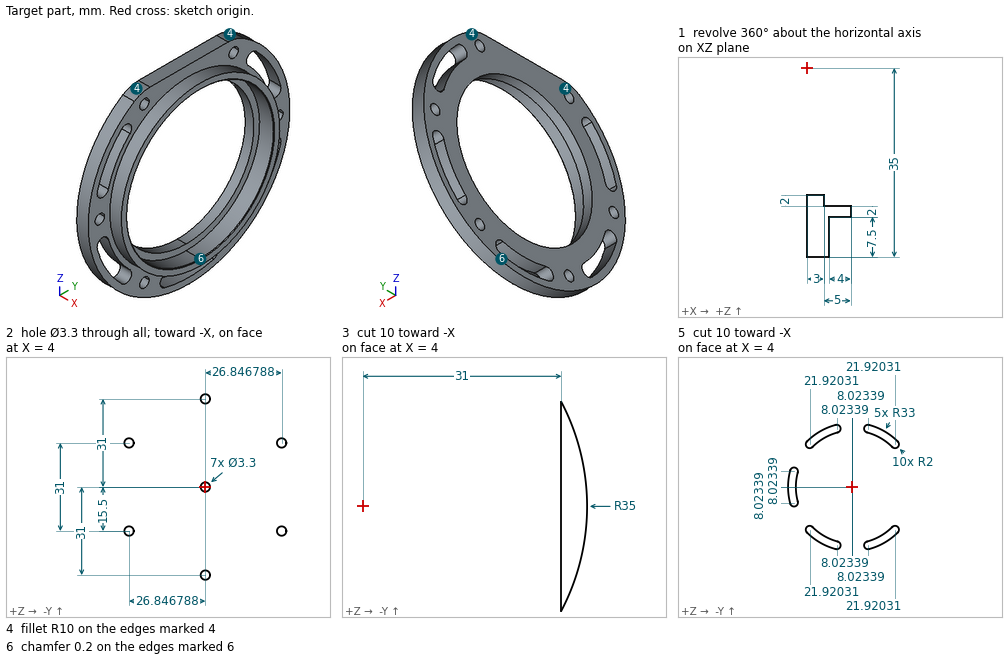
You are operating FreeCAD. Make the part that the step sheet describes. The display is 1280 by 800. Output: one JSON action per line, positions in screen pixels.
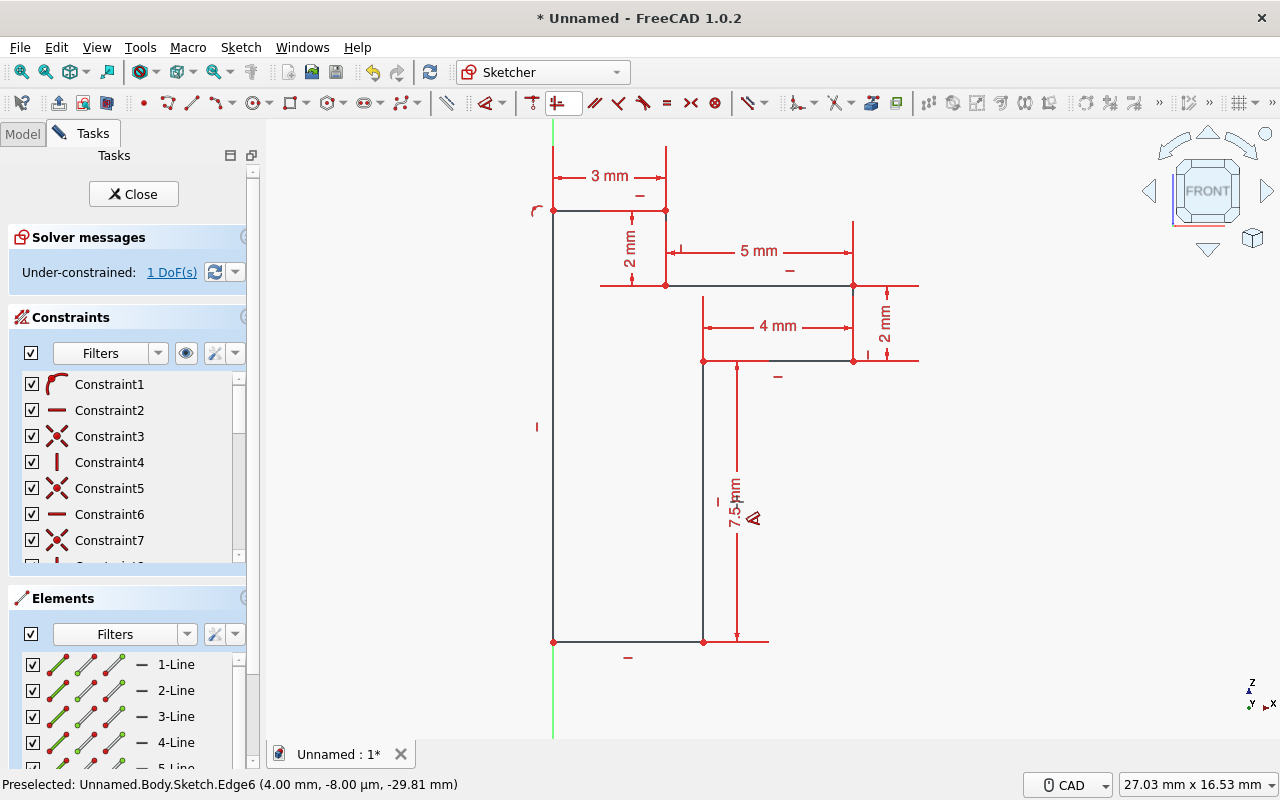
{"action": "left_click", "coordinate": [703, 642]}
{"action": "left_click", "coordinate": [519, 395]}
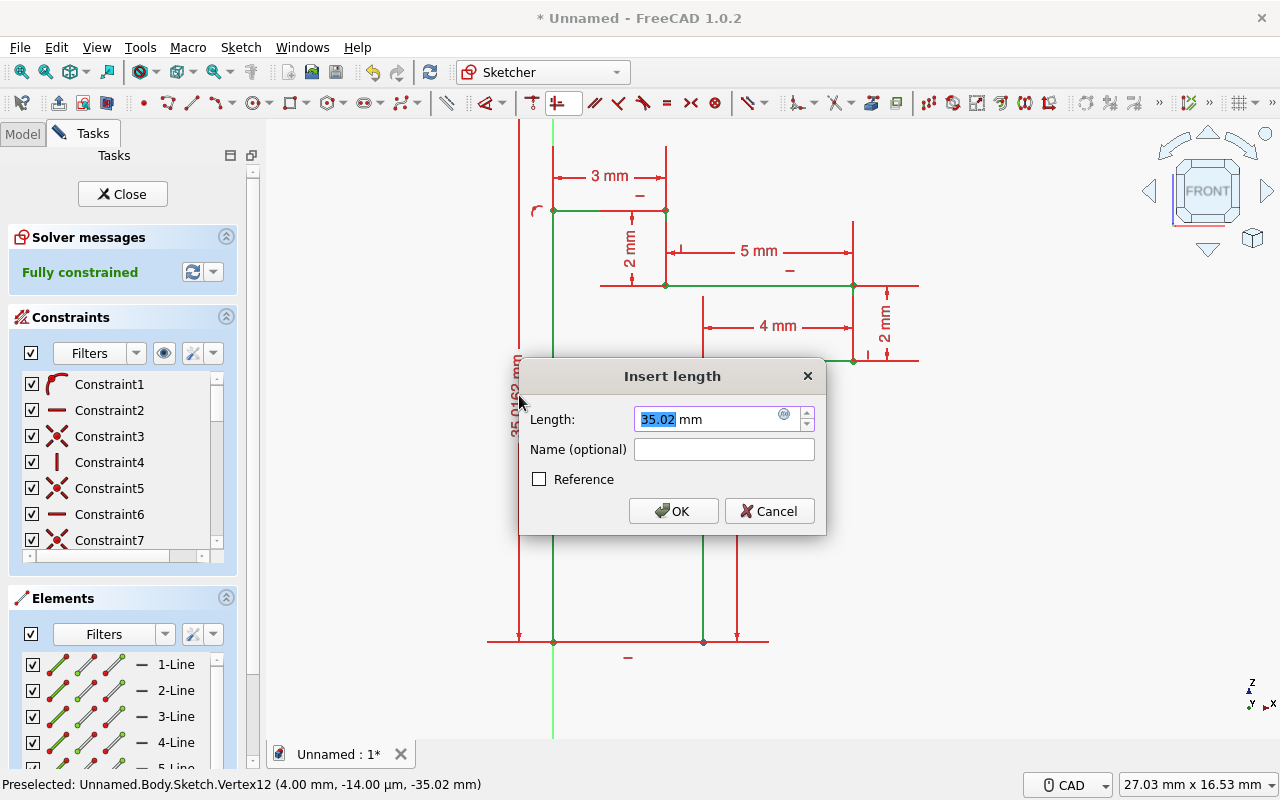
{"action": "type", "text": "35"}
{"action": "key", "text": "Return"}
{"action": "key", "text": "Escape"}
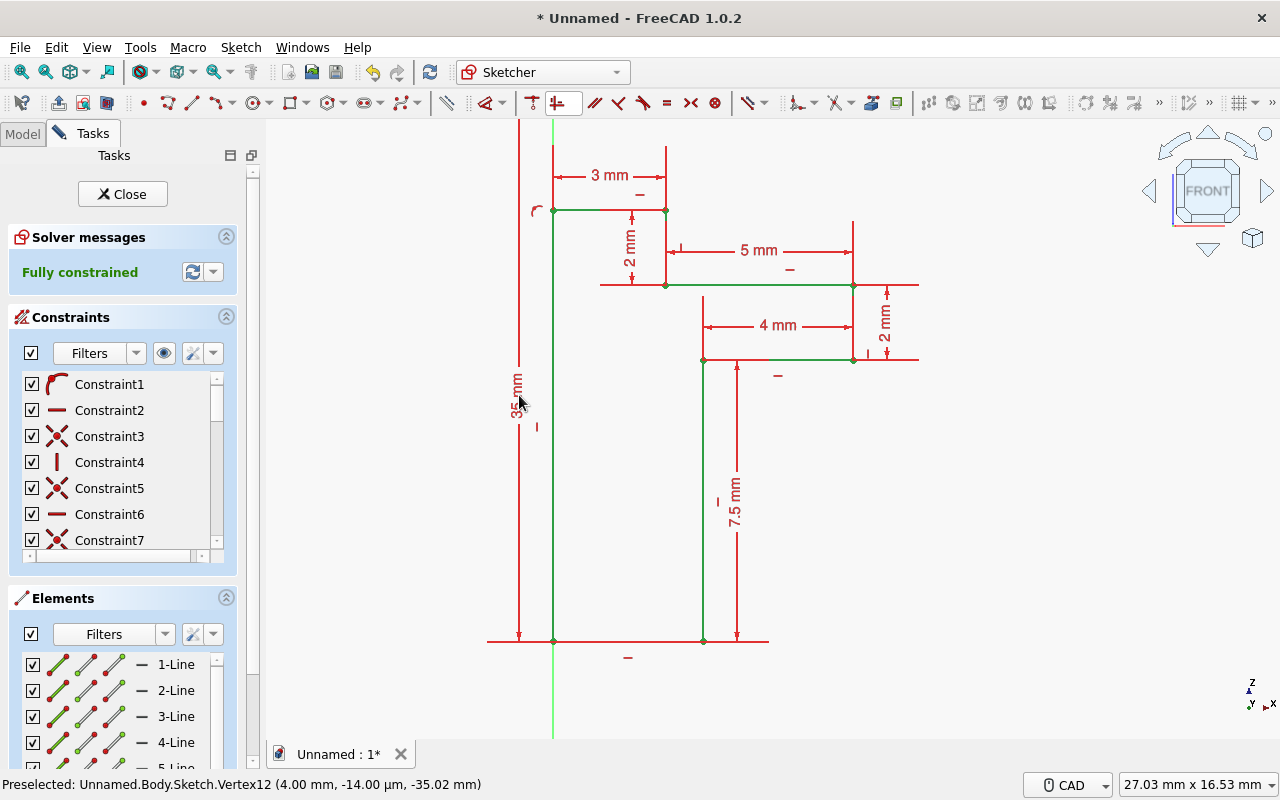
{"action": "left_click", "coordinate": [123, 194]}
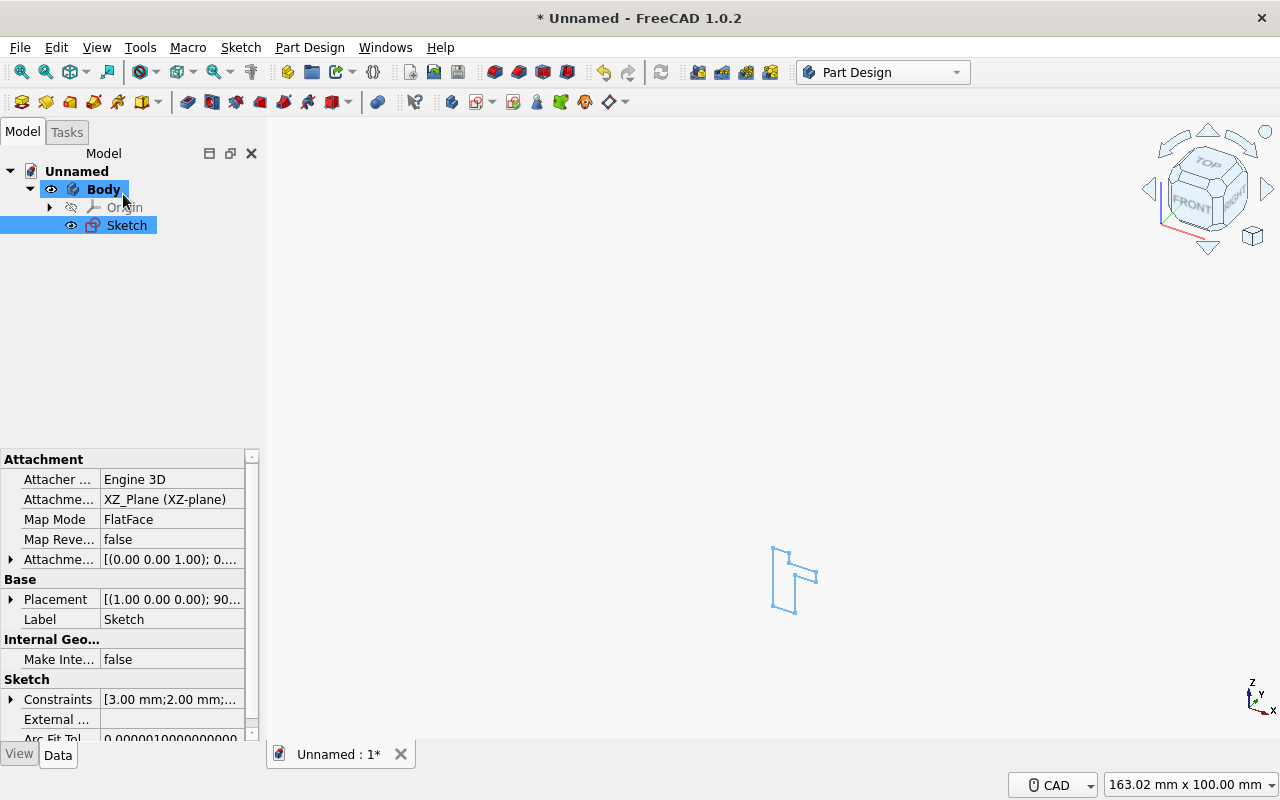
{"action": "left_click", "coordinate": [46, 102]}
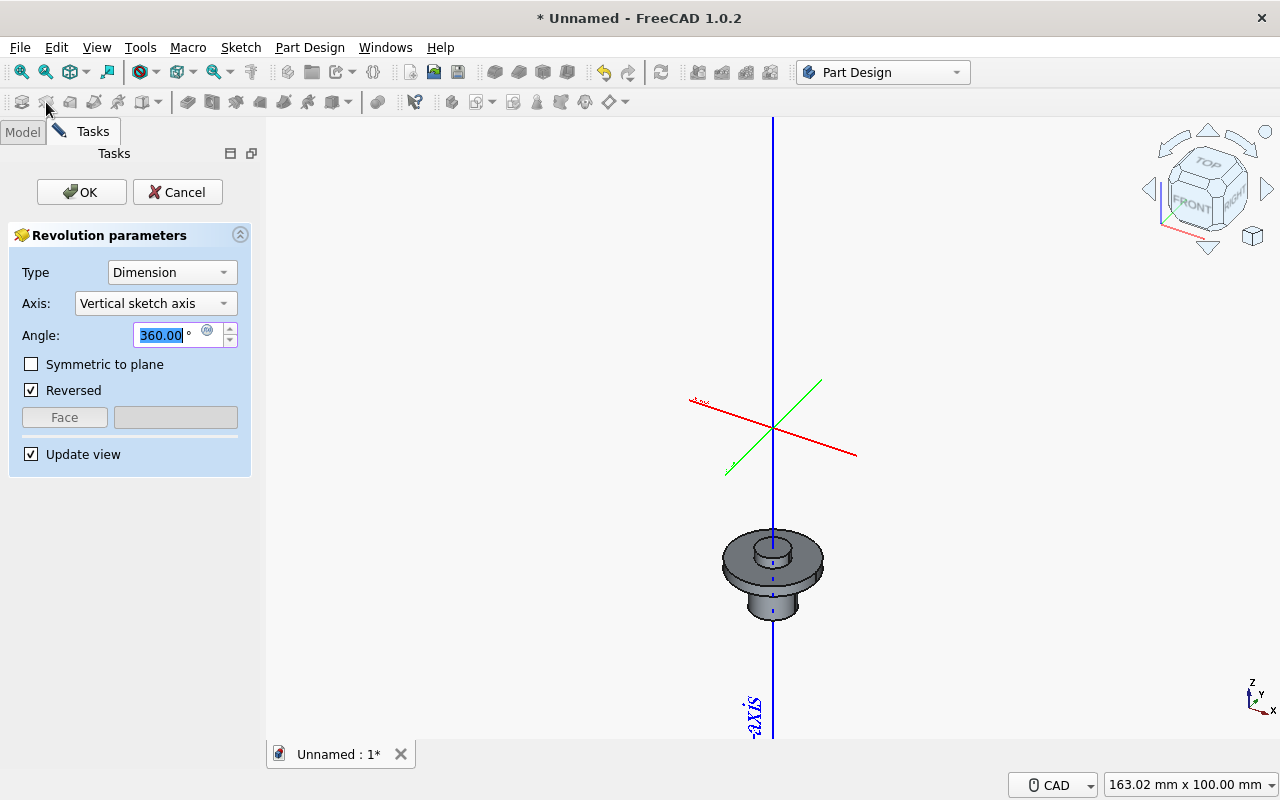
{"action": "left_click", "coordinate": [156, 304]}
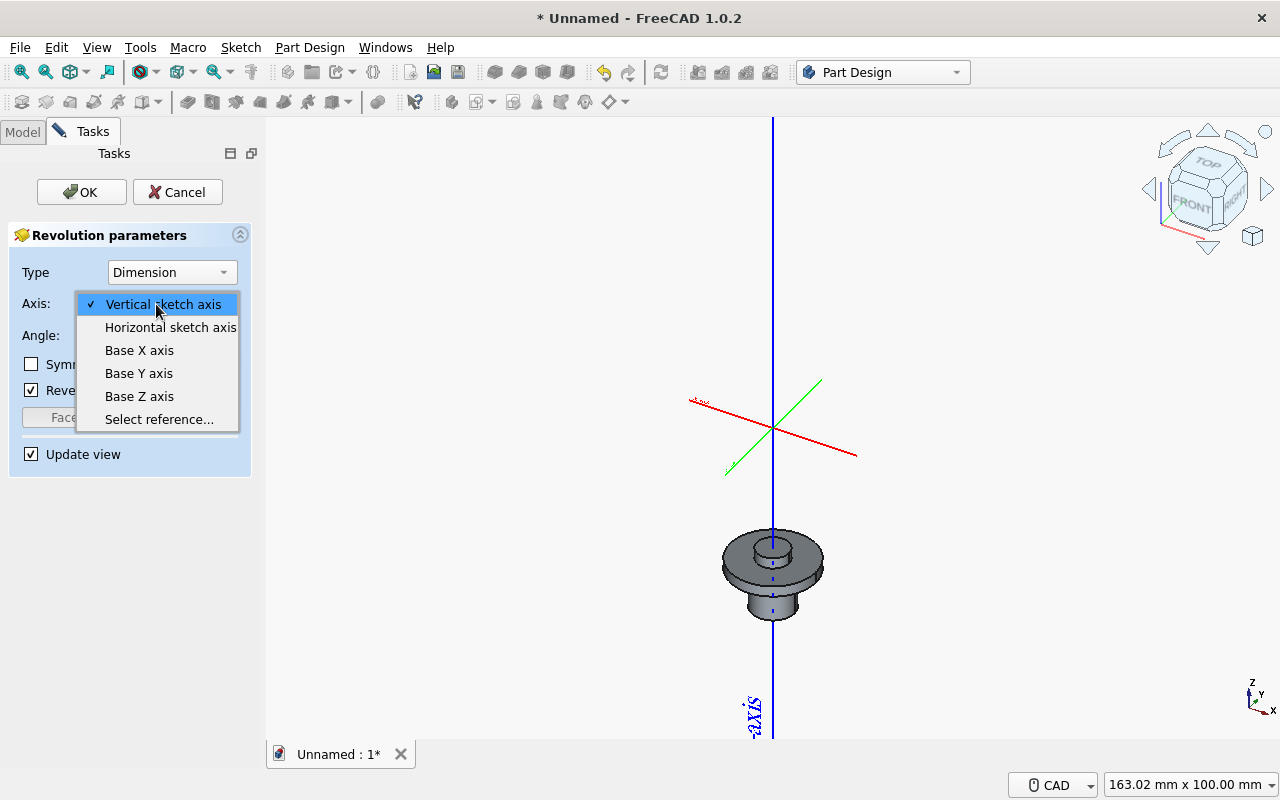
{"action": "left_click", "coordinate": [156, 328]}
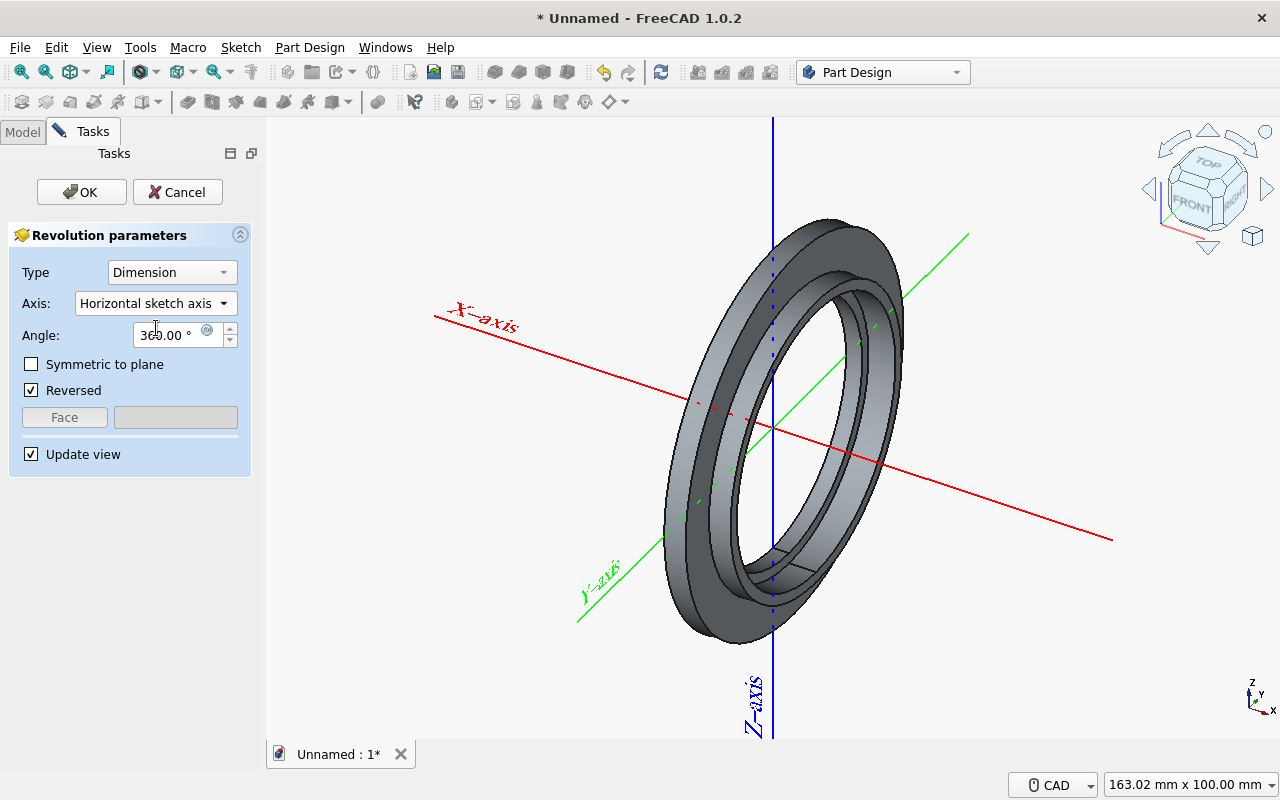
{"action": "left_click", "coordinate": [82, 192]}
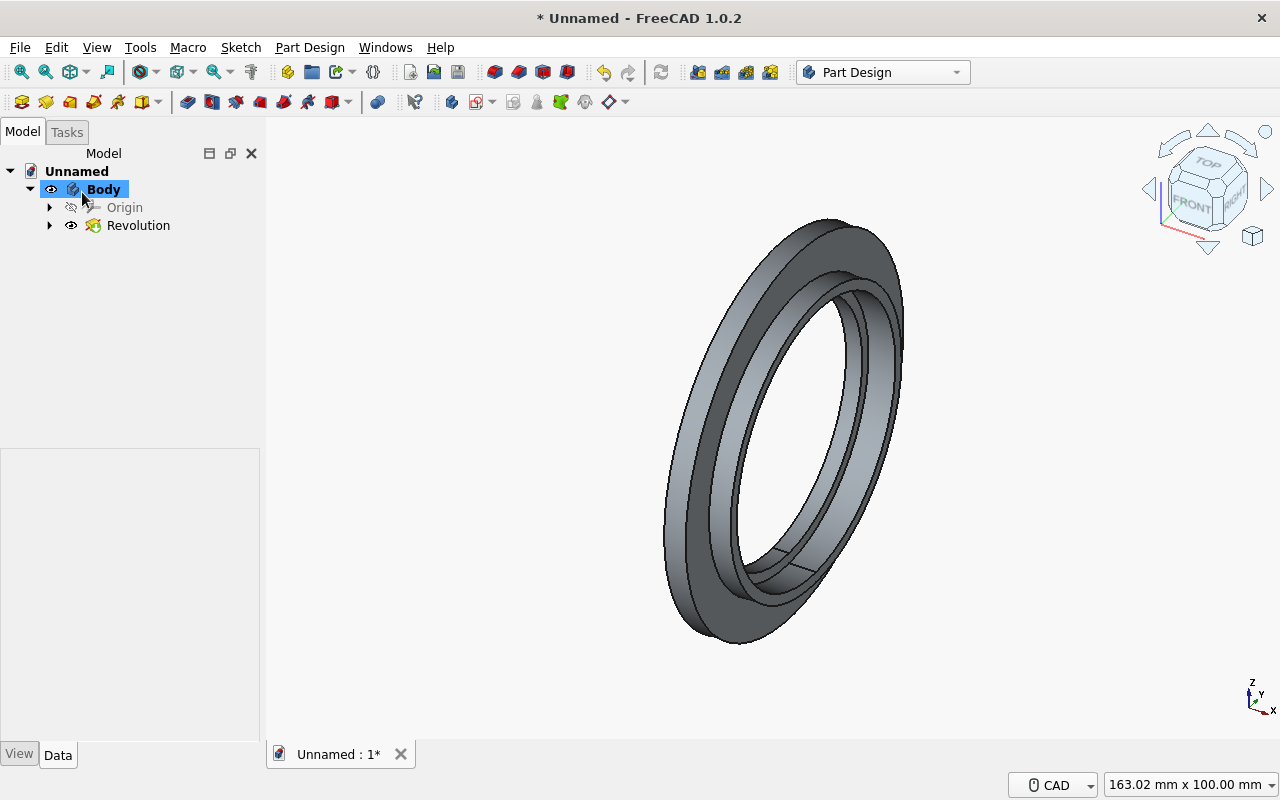
{"action": "left_click", "coordinate": [701, 476]}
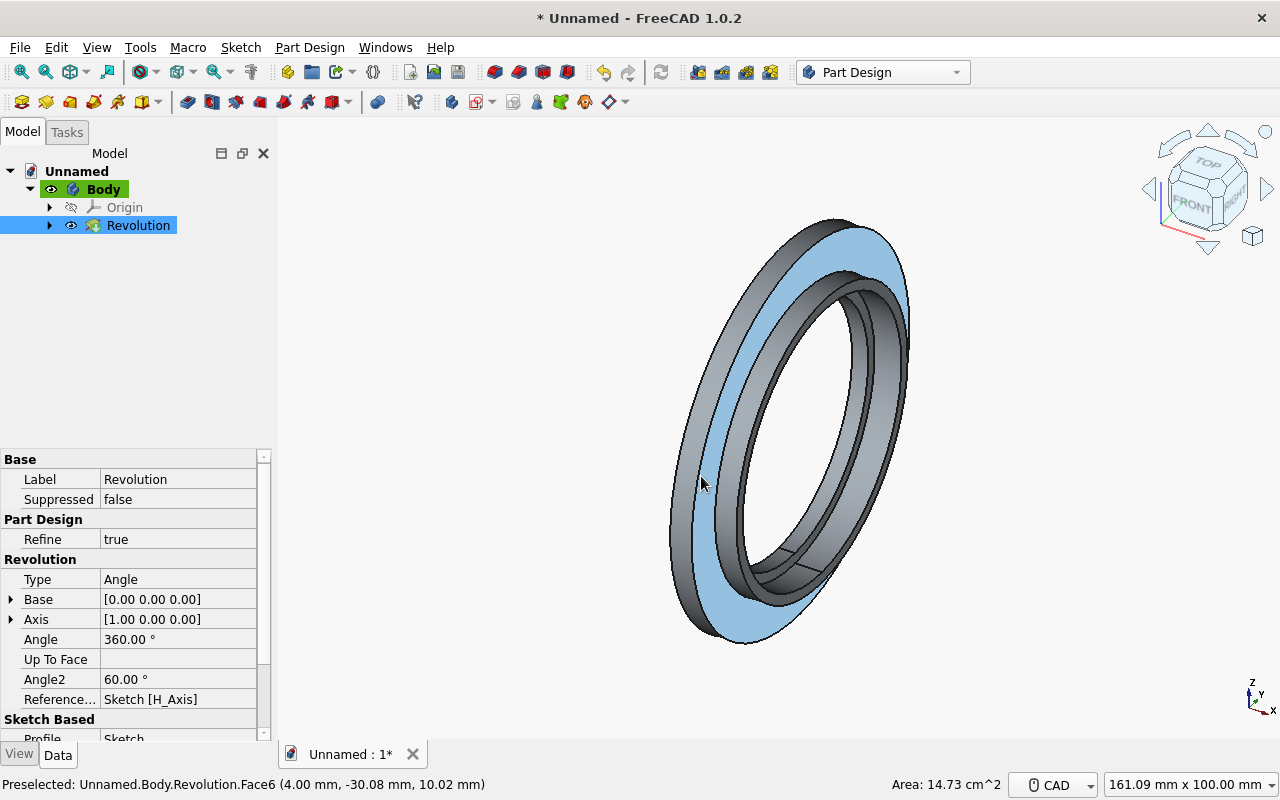
{"action": "left_click", "coordinate": [476, 102]}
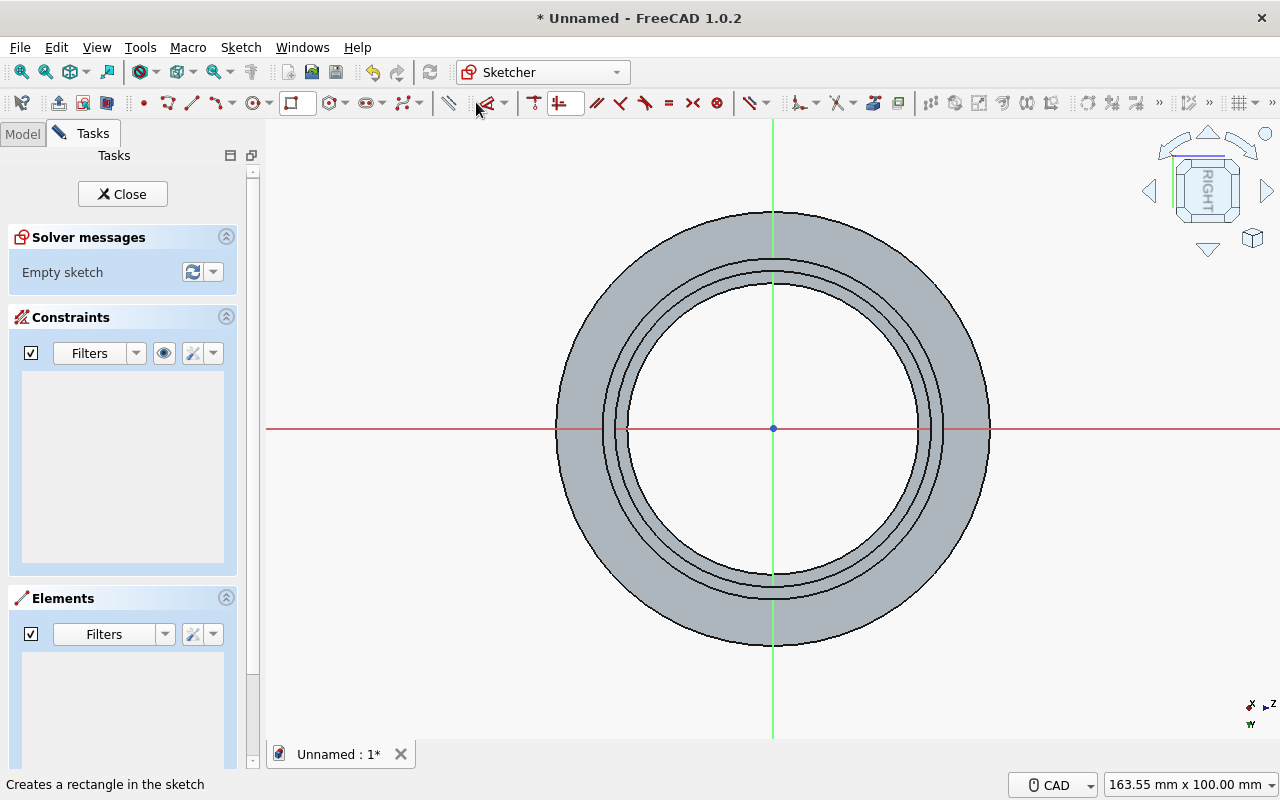
{"action": "left_click", "coordinate": [108, 104]}